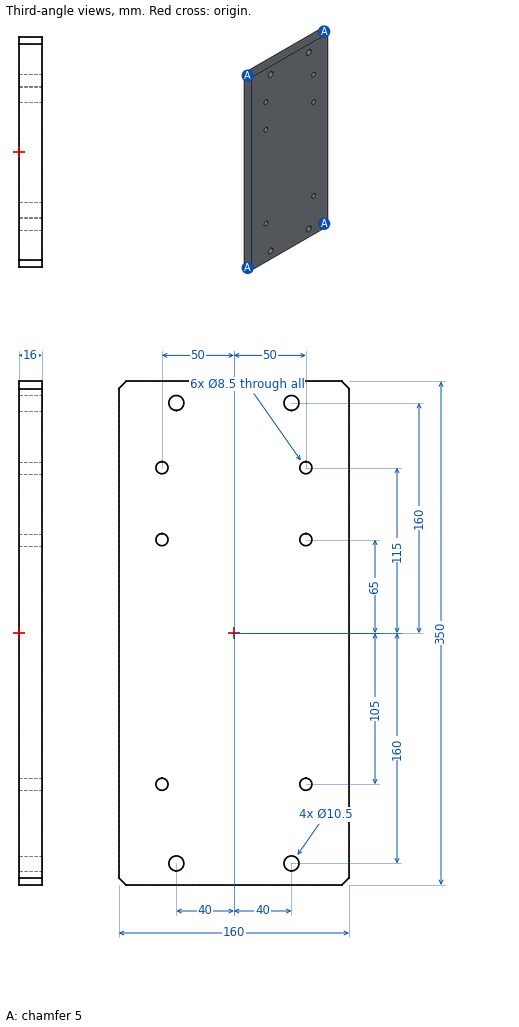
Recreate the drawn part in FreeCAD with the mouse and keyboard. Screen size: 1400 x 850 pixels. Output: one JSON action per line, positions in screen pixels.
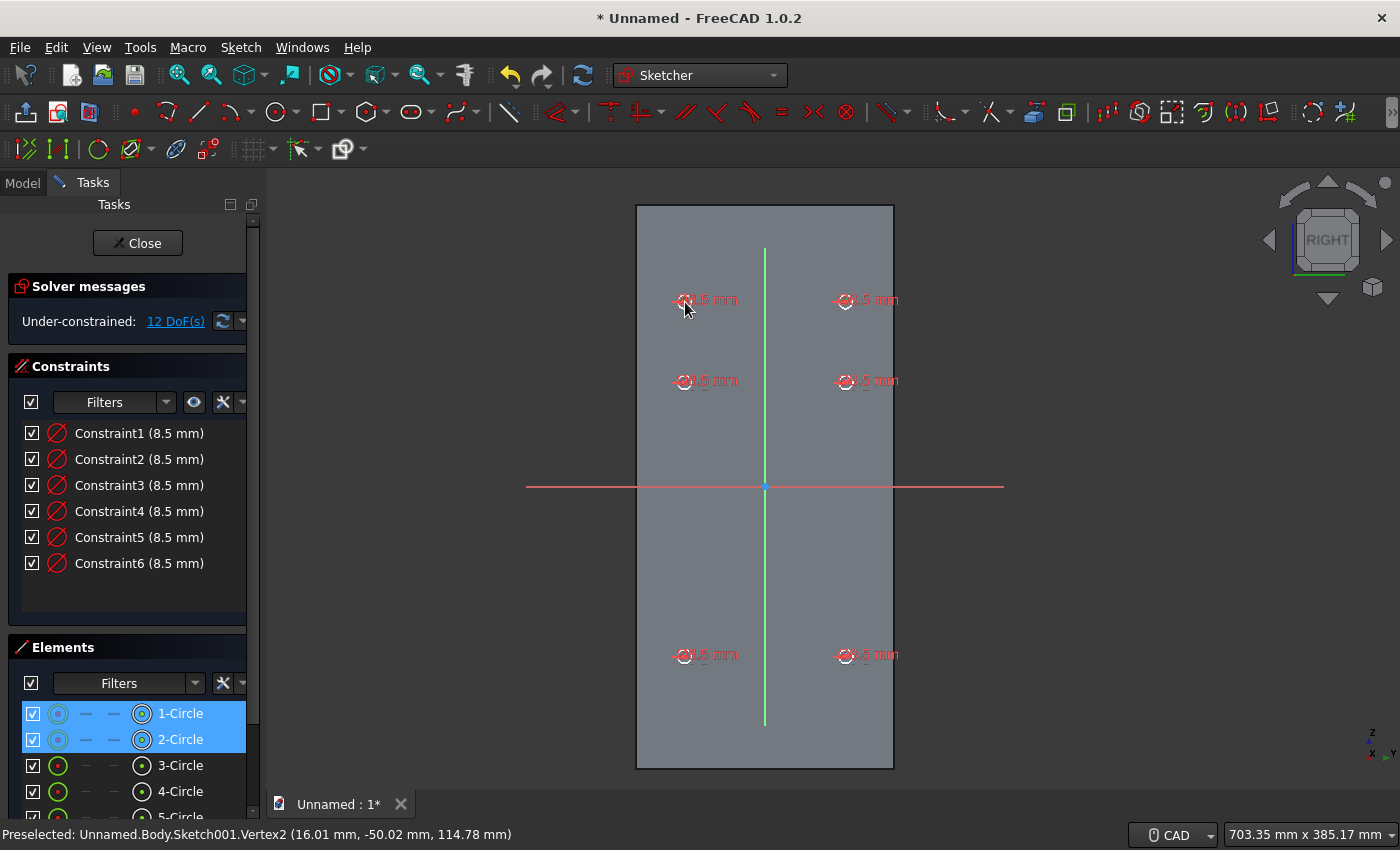
{"action": "key", "text": "h"}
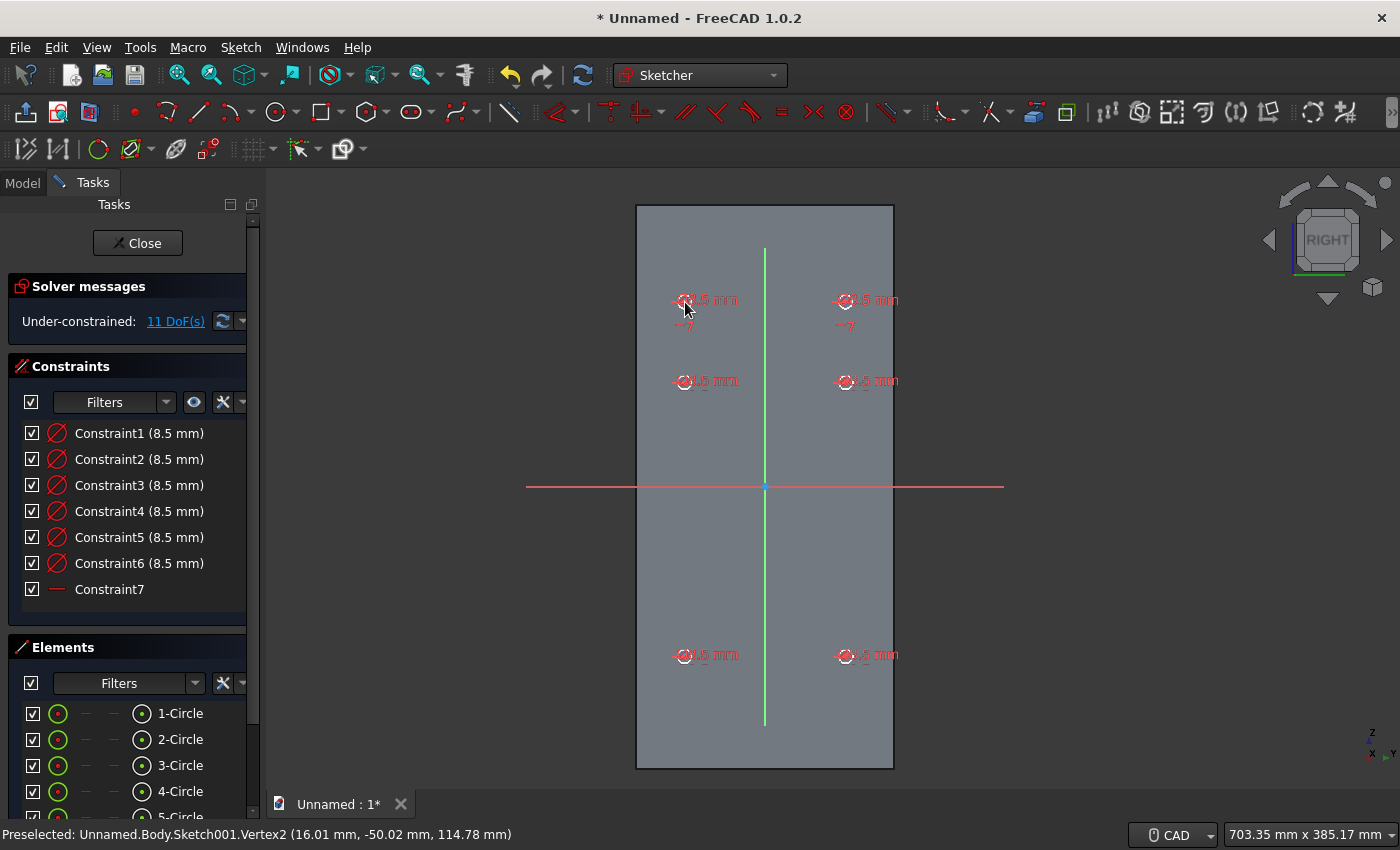
{"action": "left_click", "coordinate": [846, 302]}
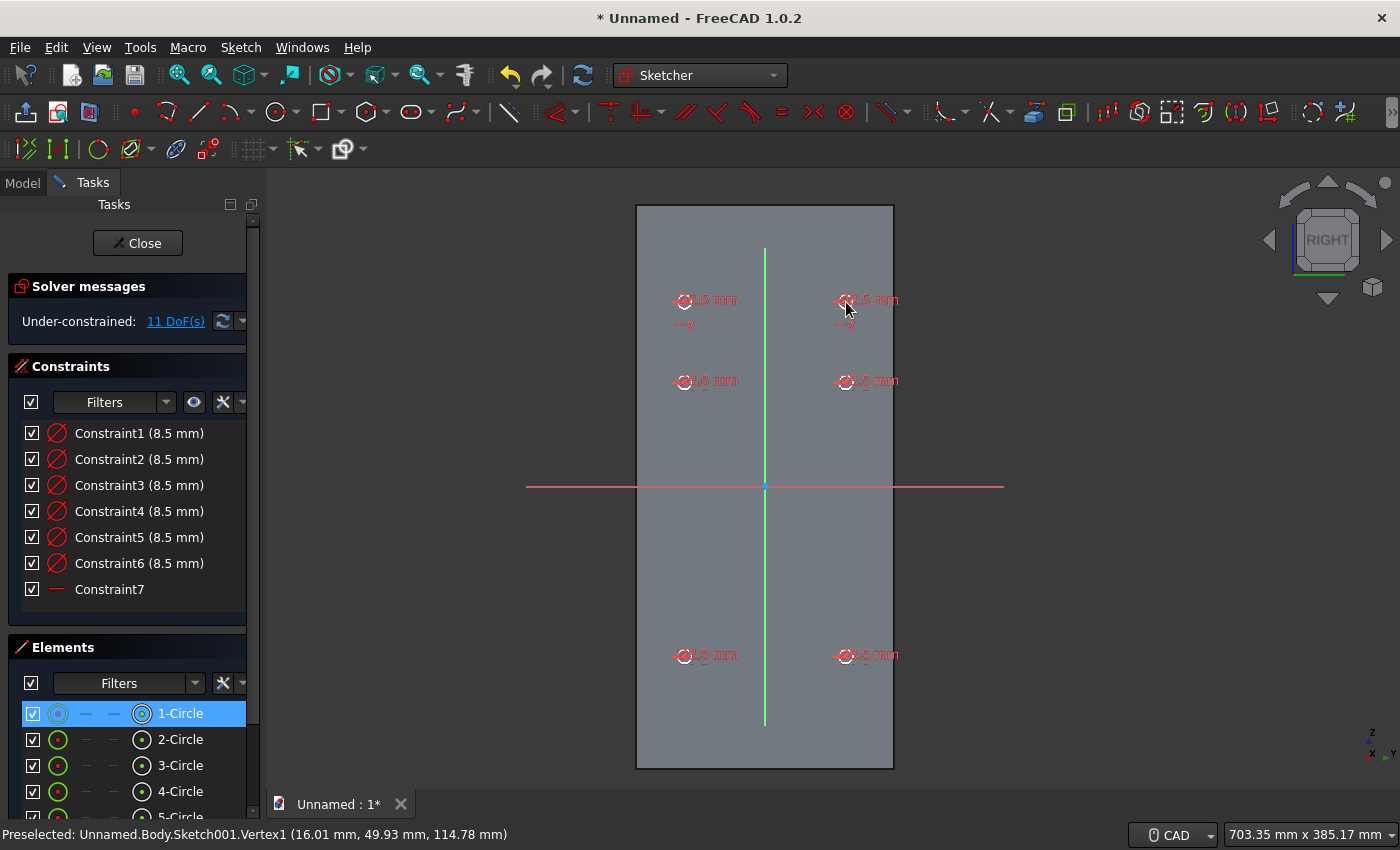
{"action": "left_click", "coordinate": [846, 657]}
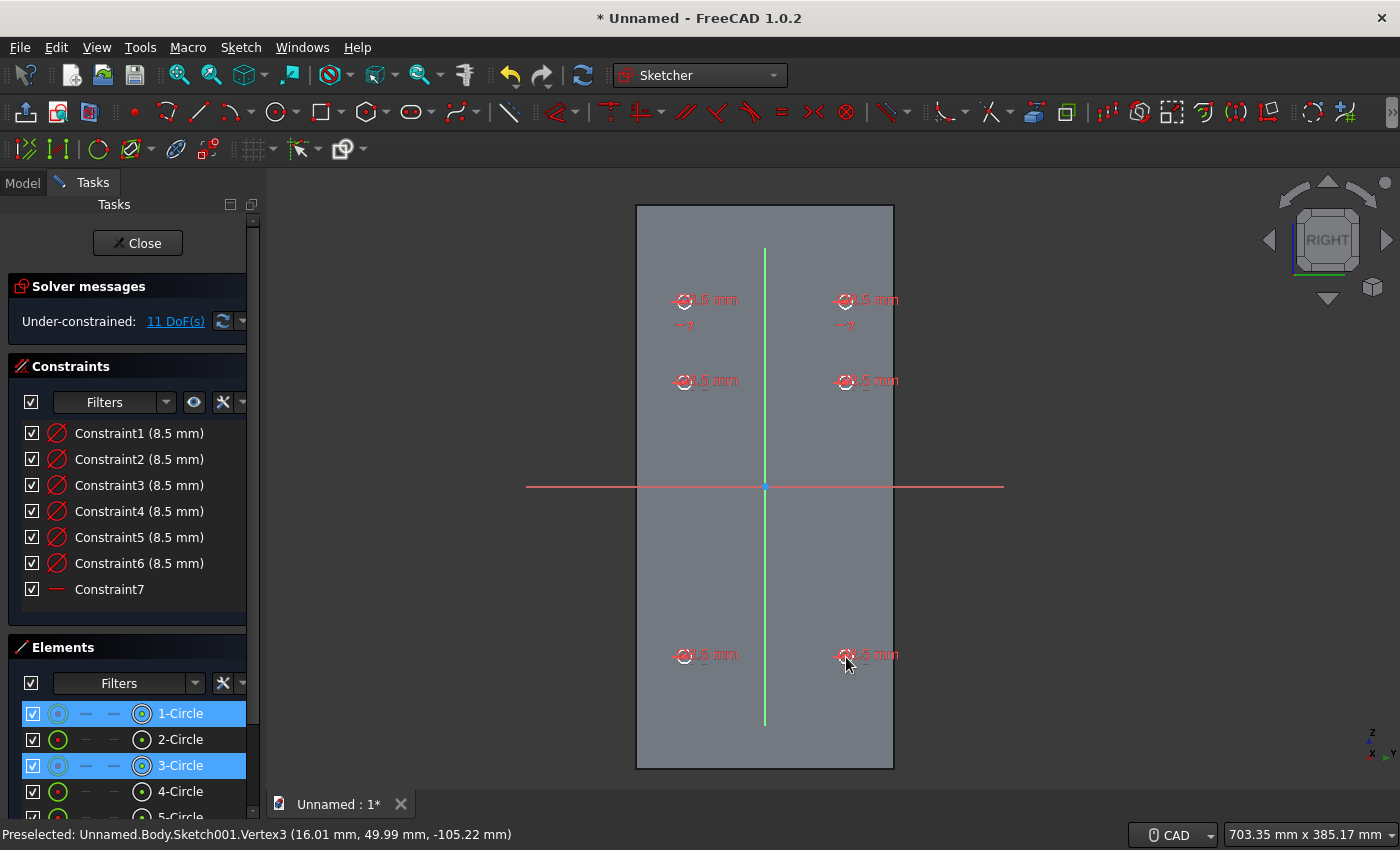
{"action": "key", "text": "v"}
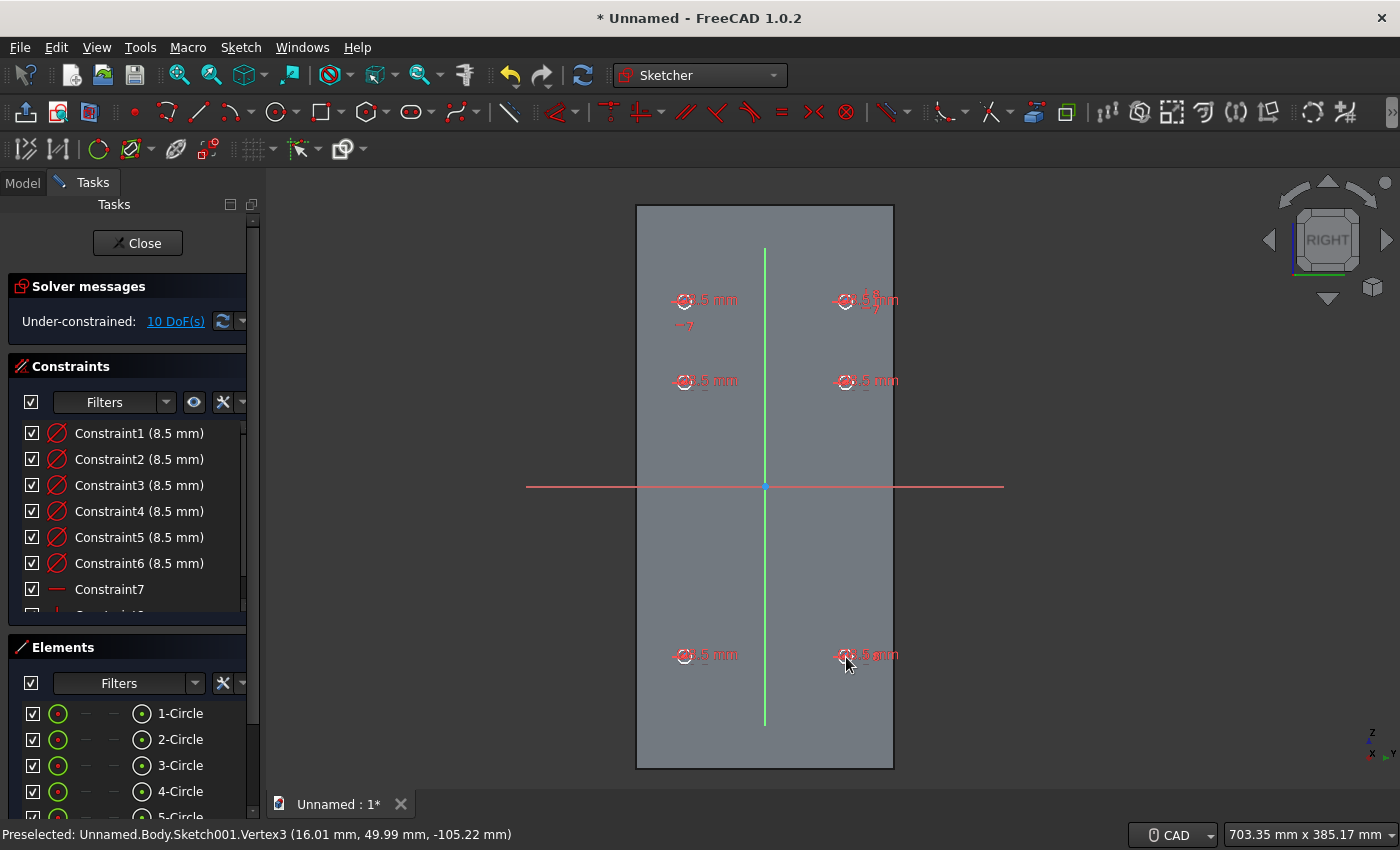
{"action": "left_click", "coordinate": [685, 302]}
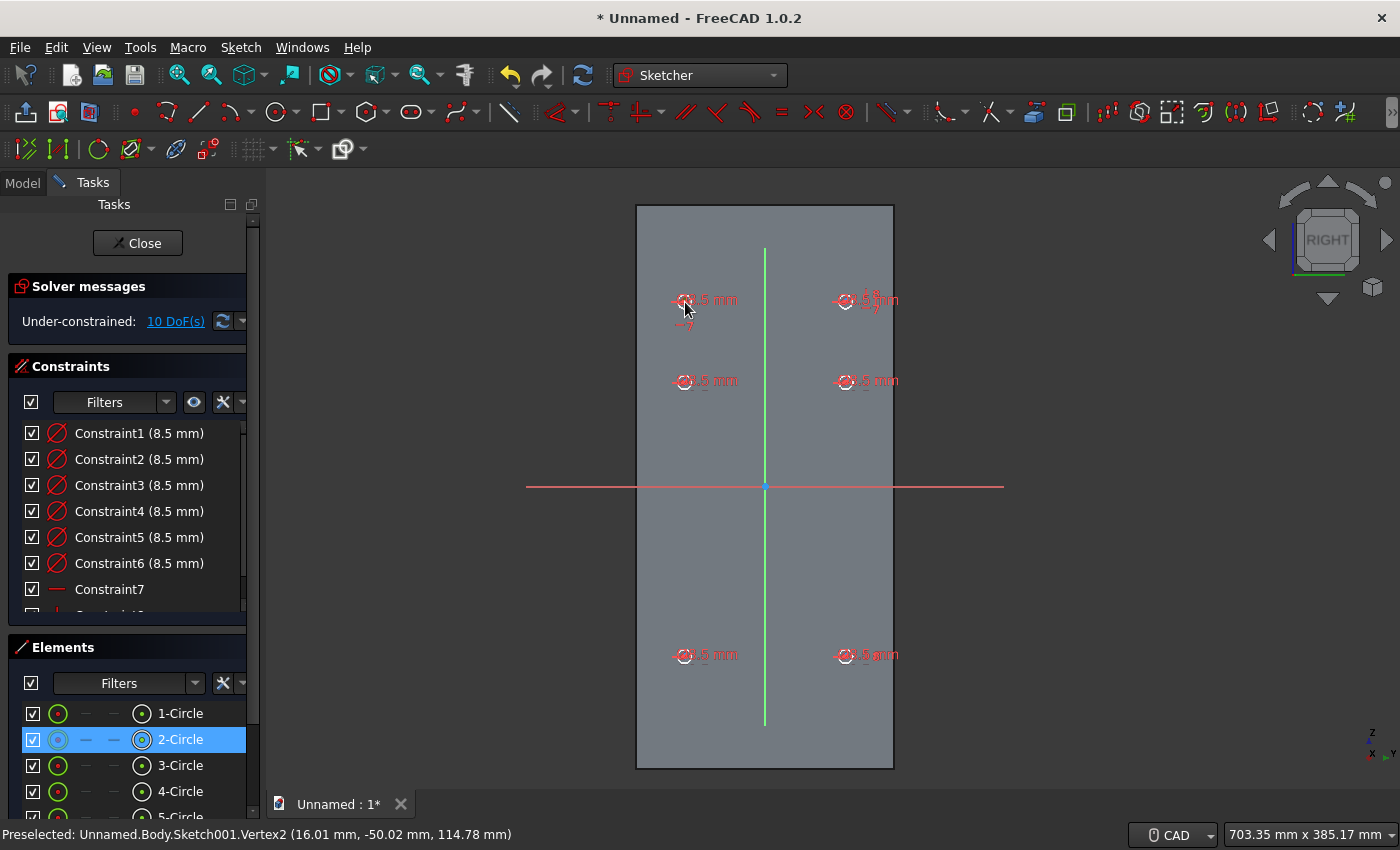
{"action": "left_click", "coordinate": [685, 657]}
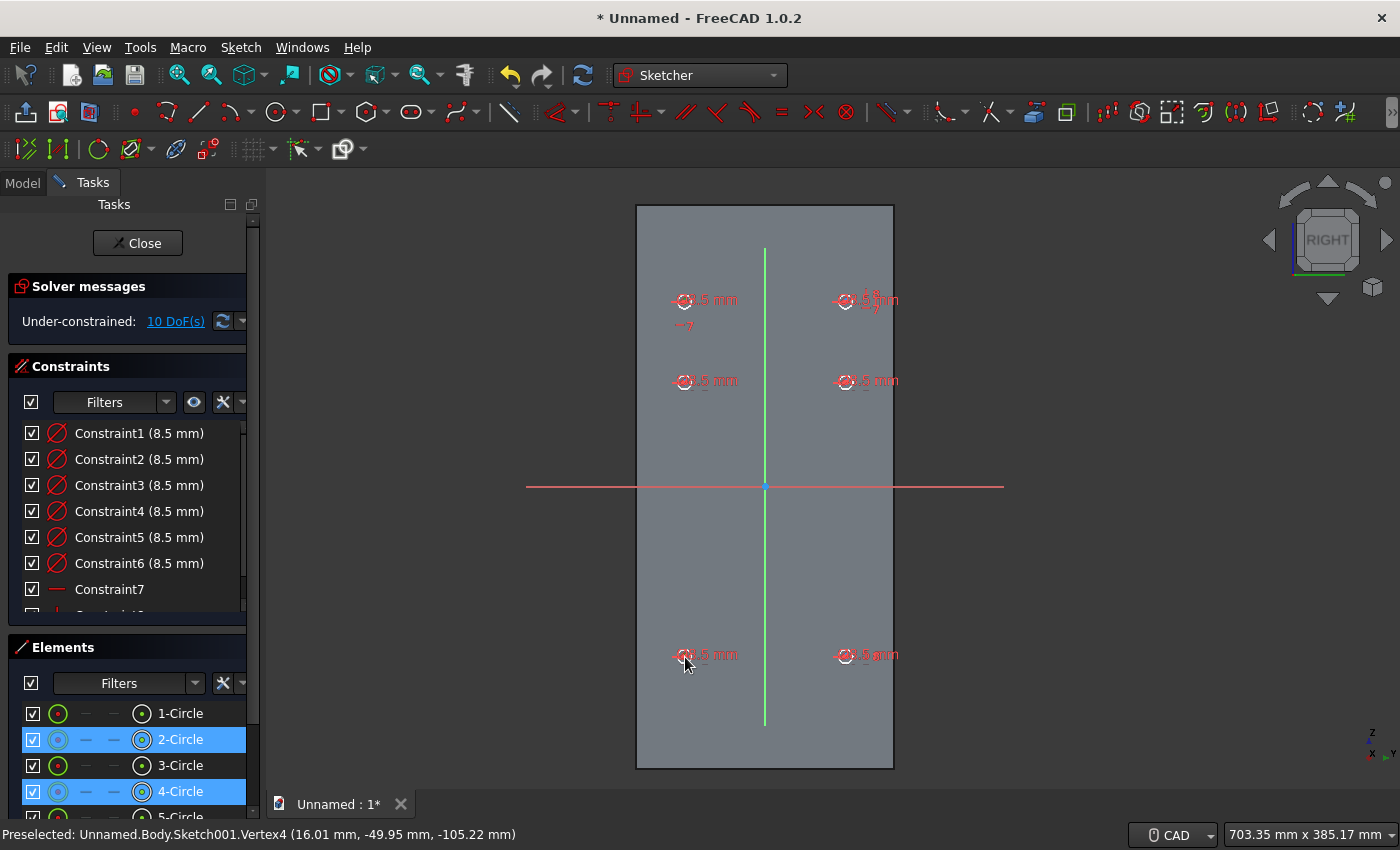
{"action": "key", "text": "v"}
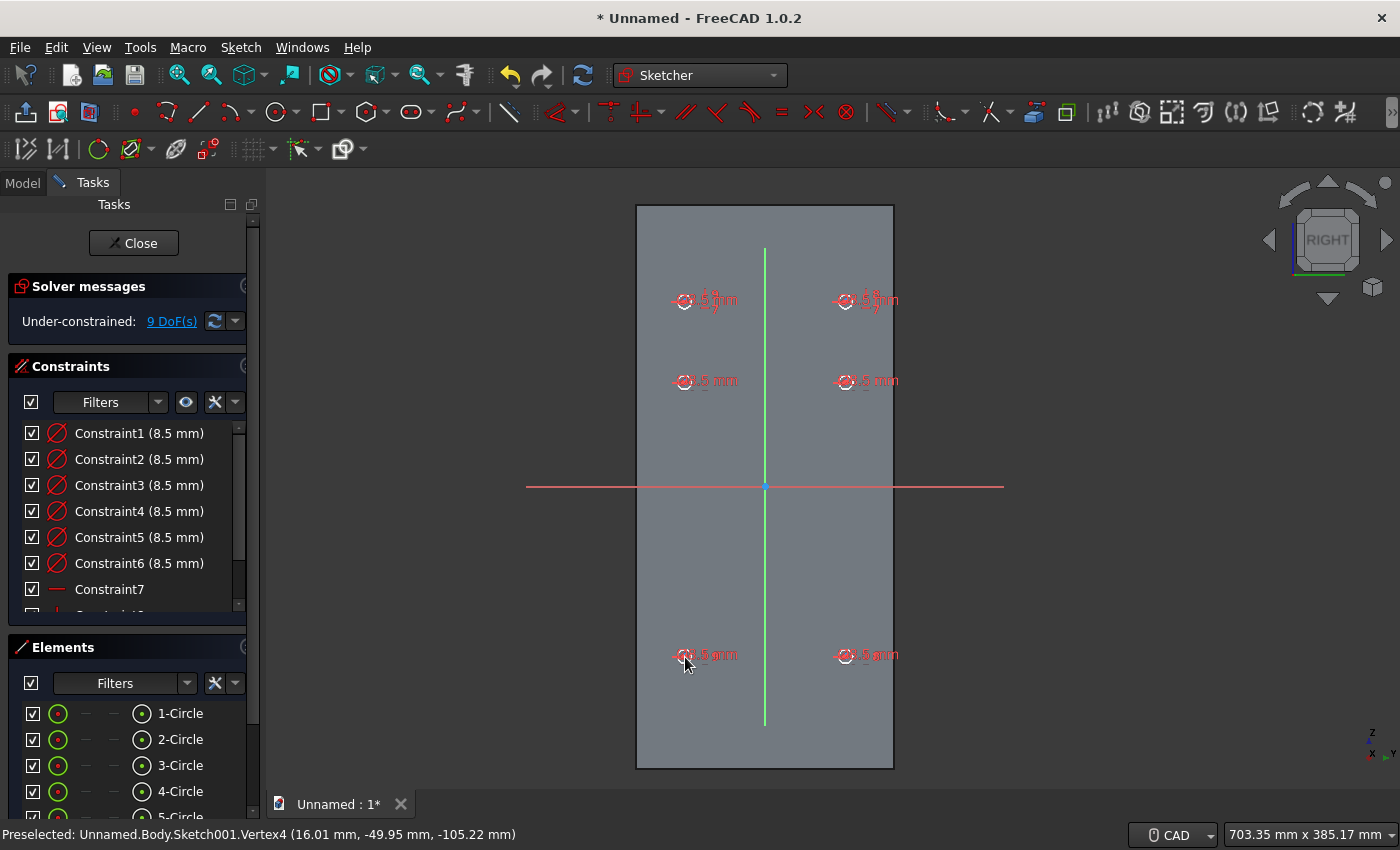
{"action": "left_click", "coordinate": [846, 657]}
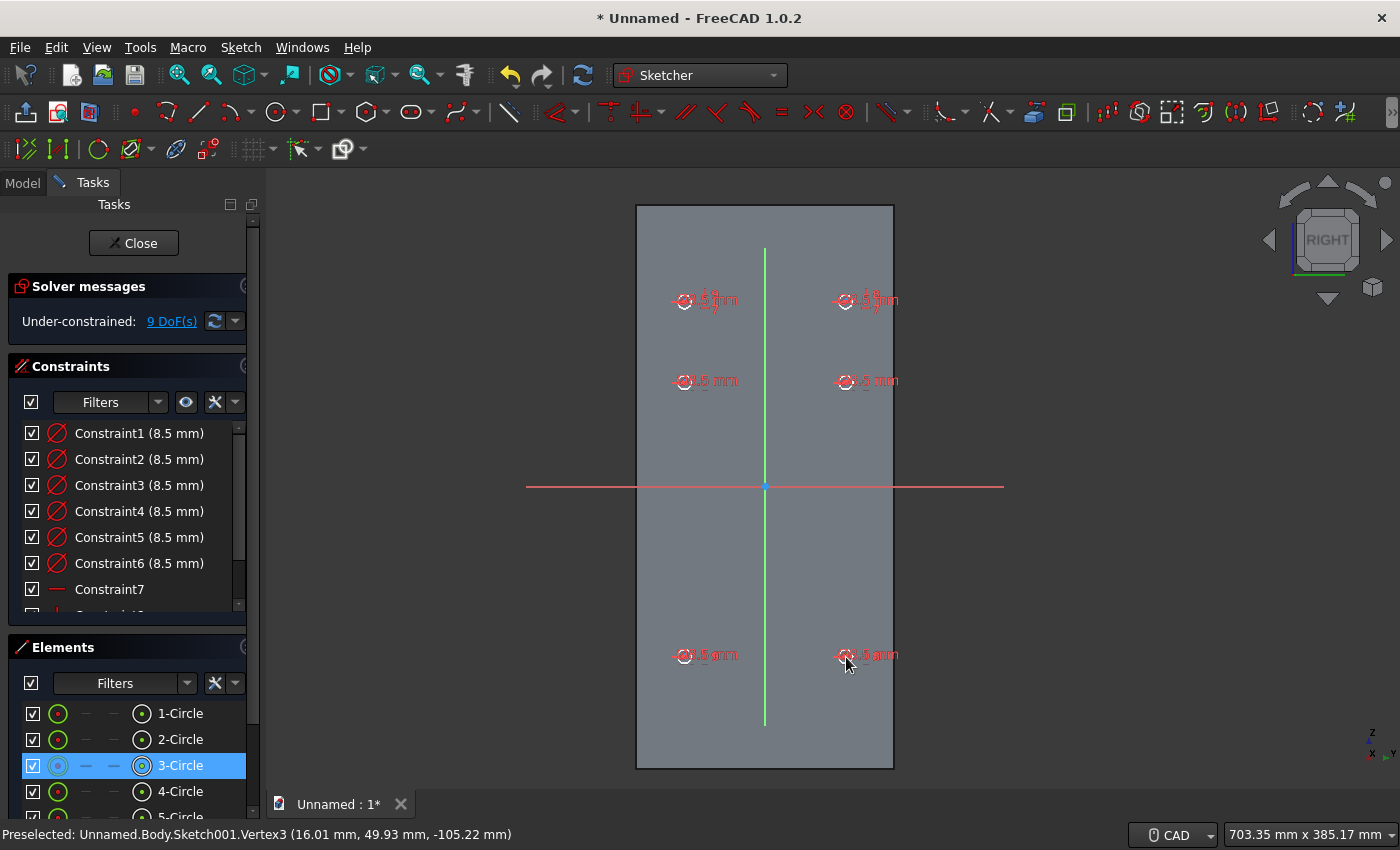
{"action": "left_click", "coordinate": [685, 657]}